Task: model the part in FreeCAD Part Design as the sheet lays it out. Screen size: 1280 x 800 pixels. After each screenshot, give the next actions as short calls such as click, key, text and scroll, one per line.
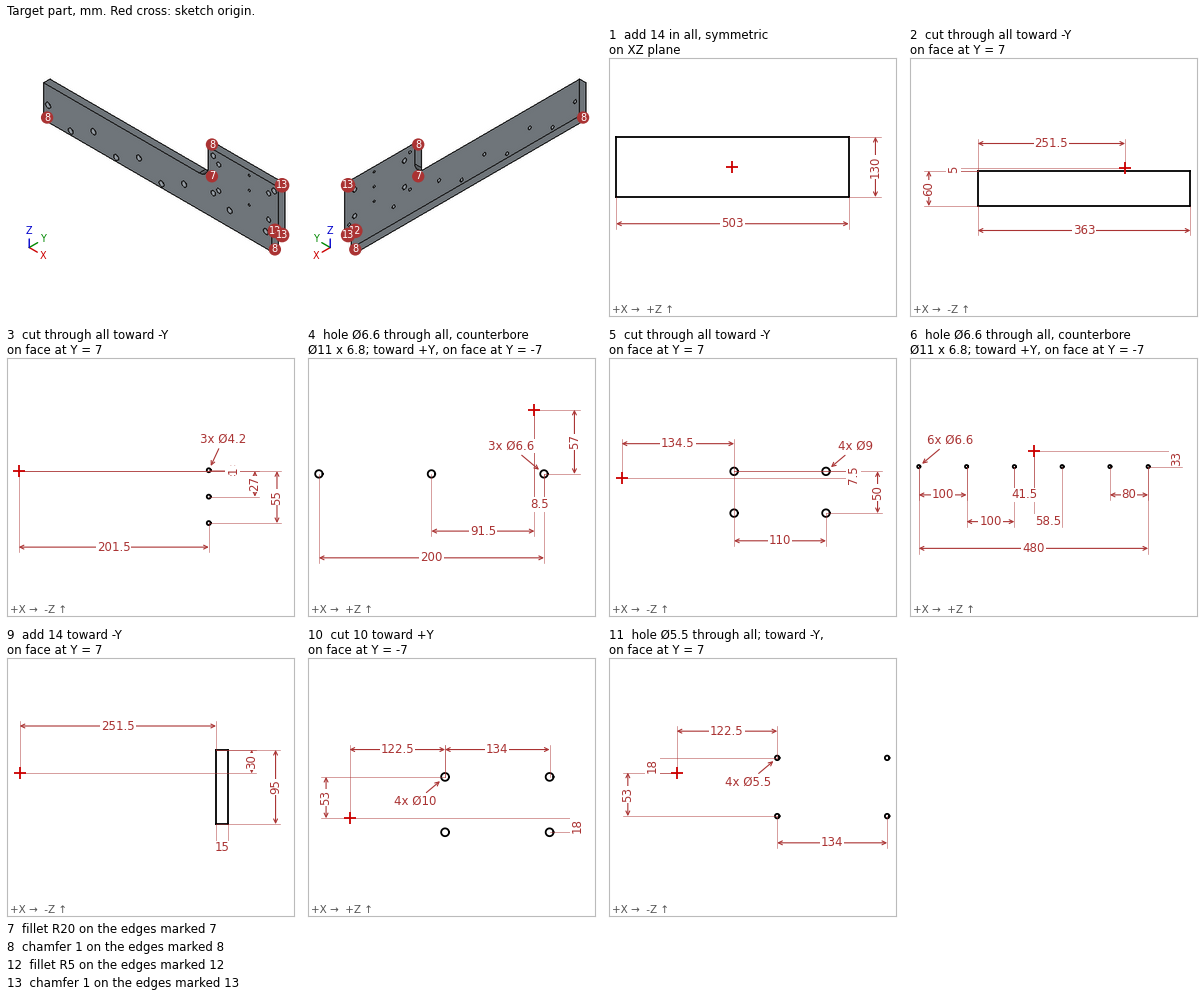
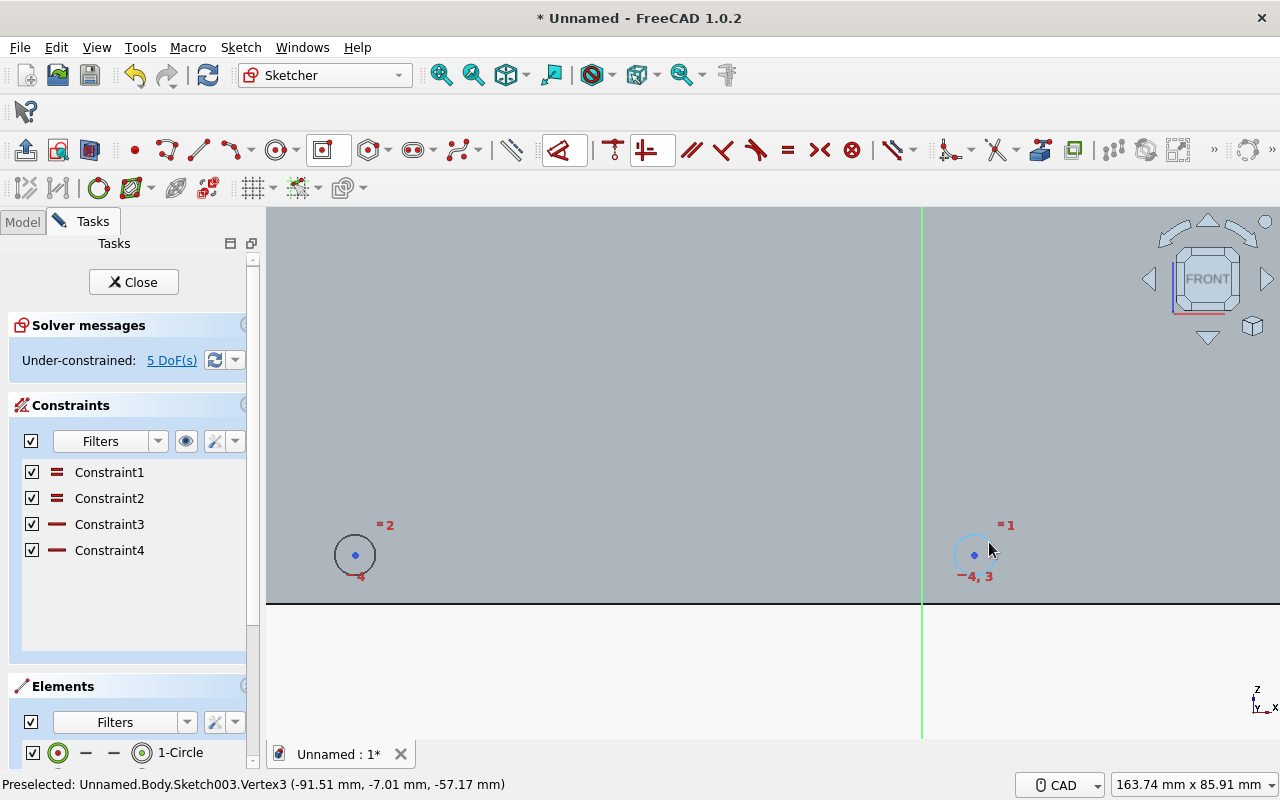
click(989, 541)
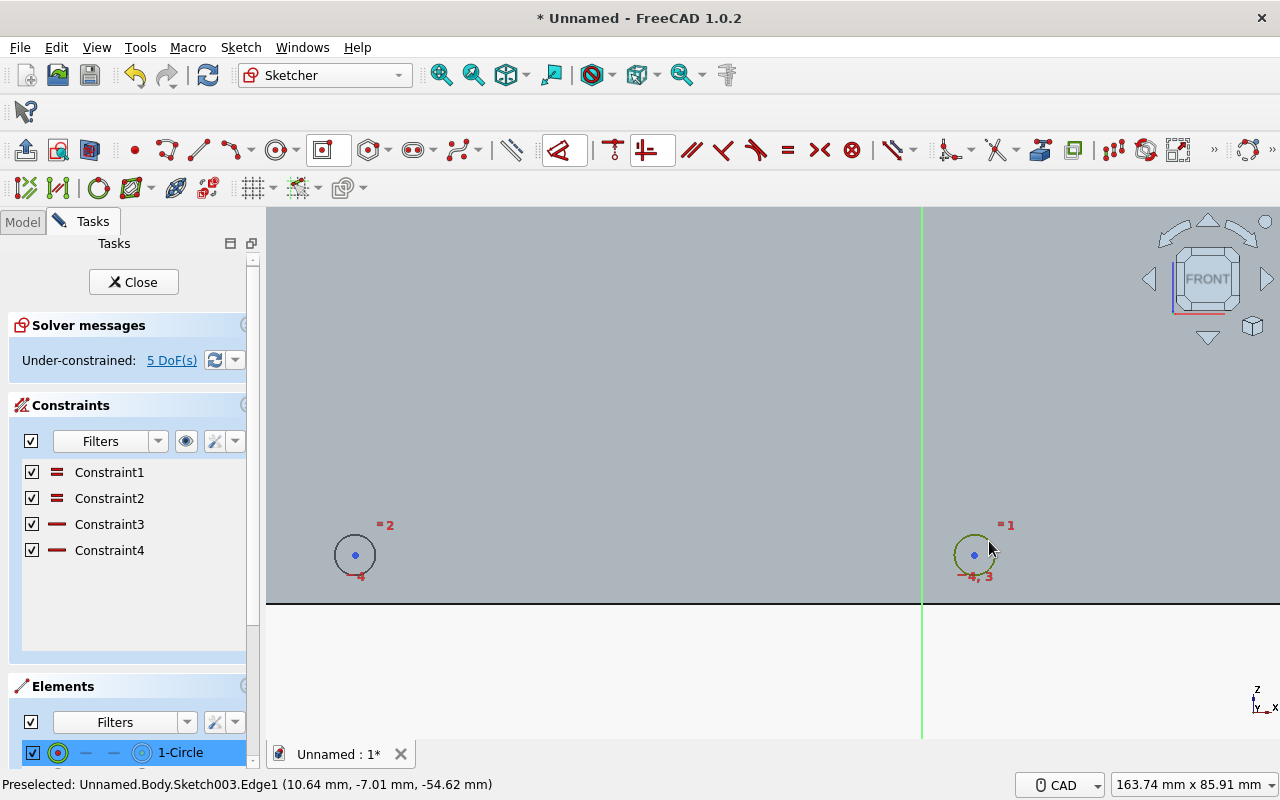
click(582, 150)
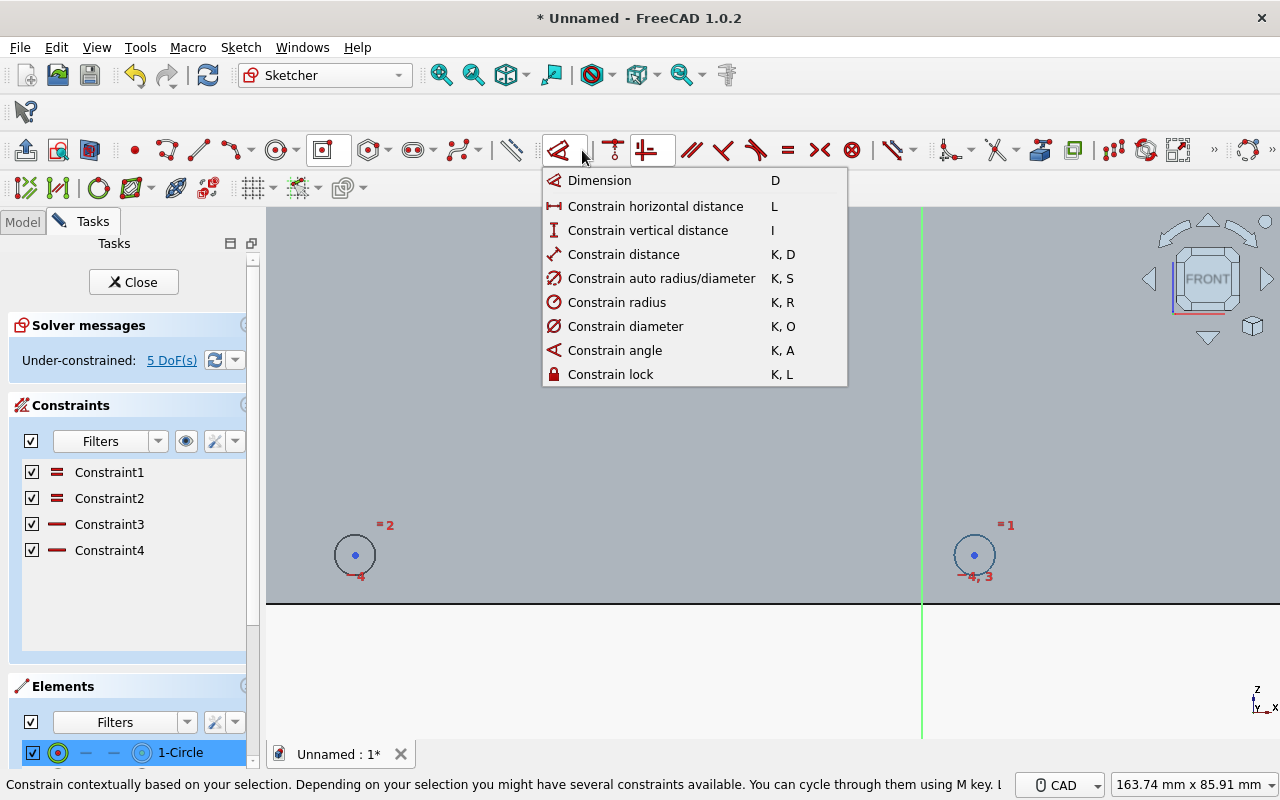
click(695, 326)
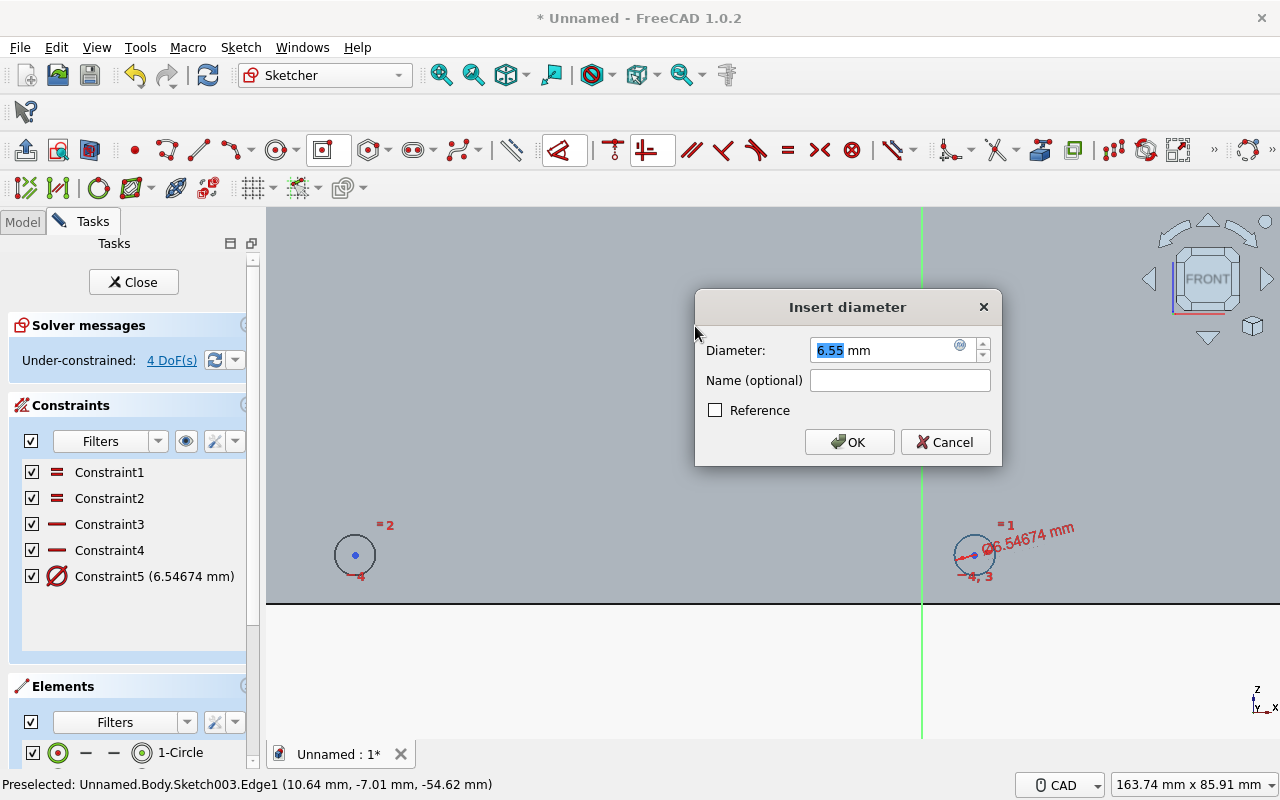
text(6.6)
key(Return)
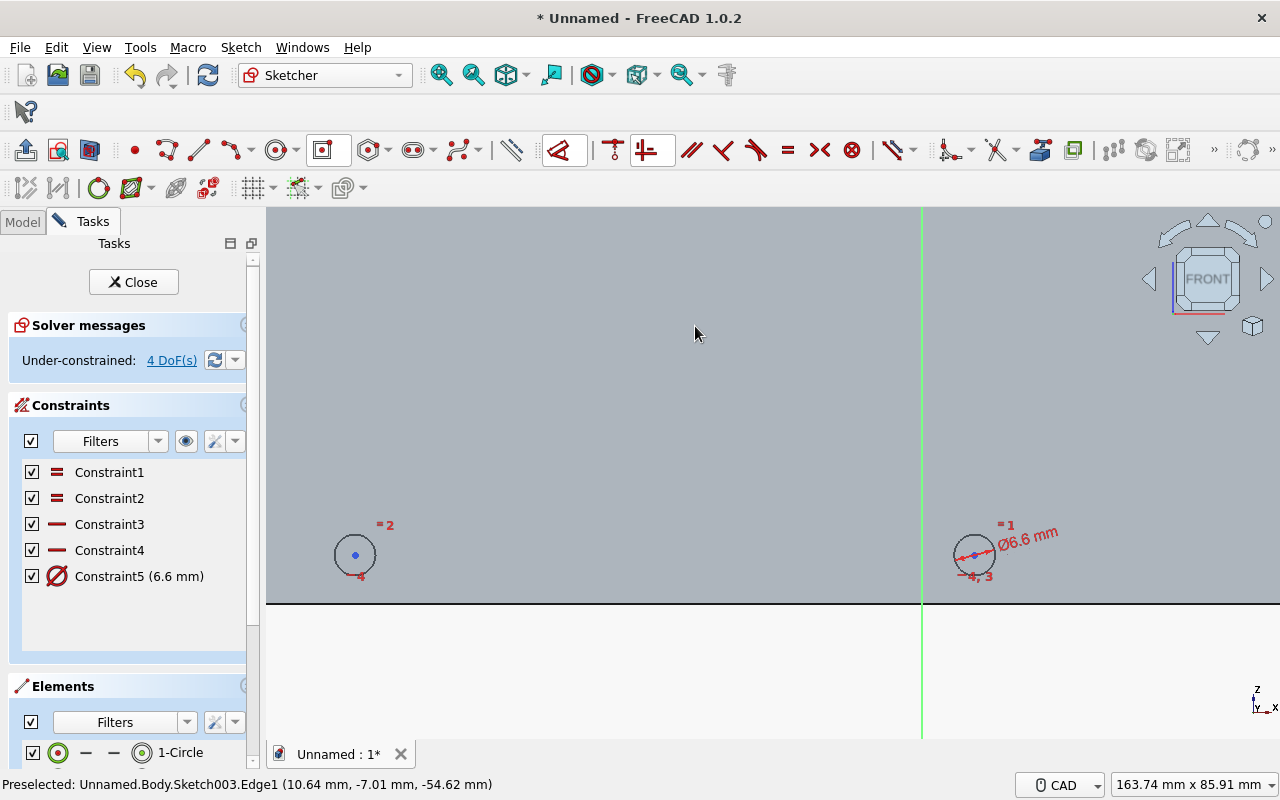
click(975, 555)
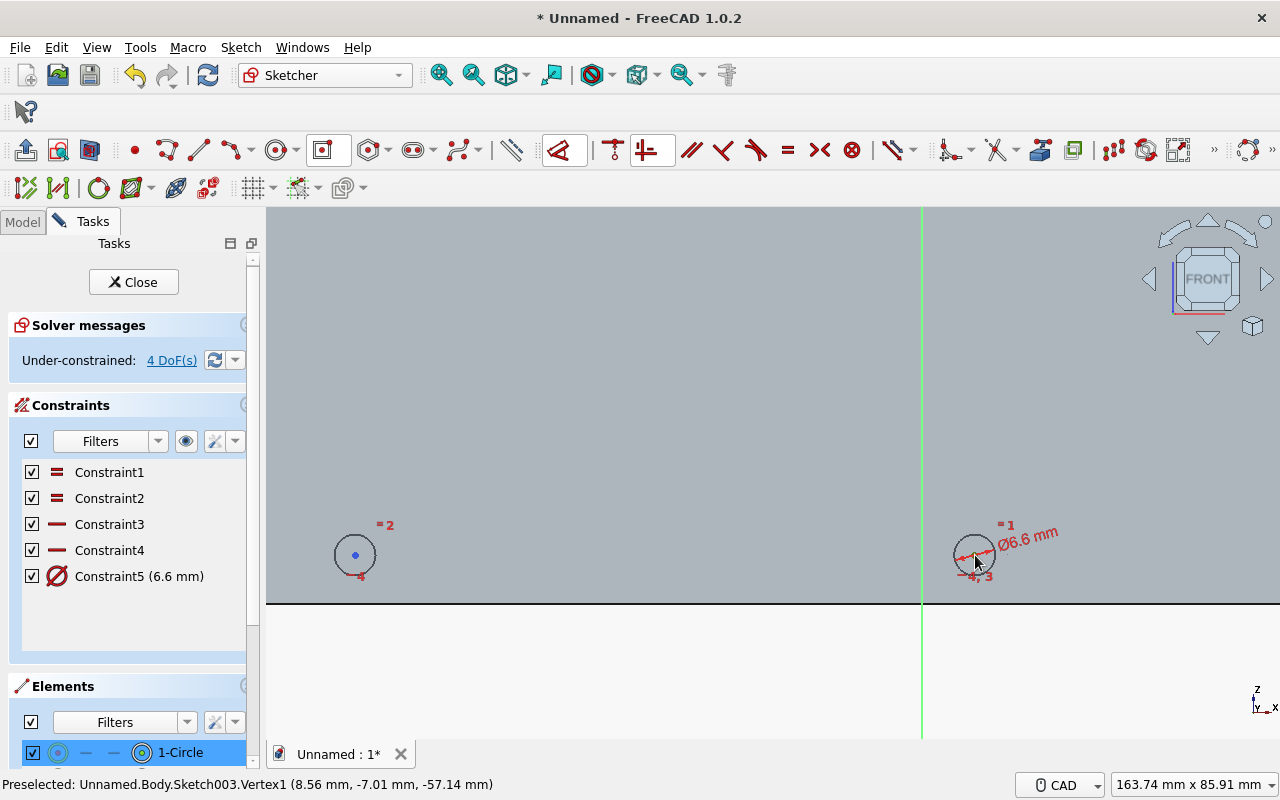
key(i)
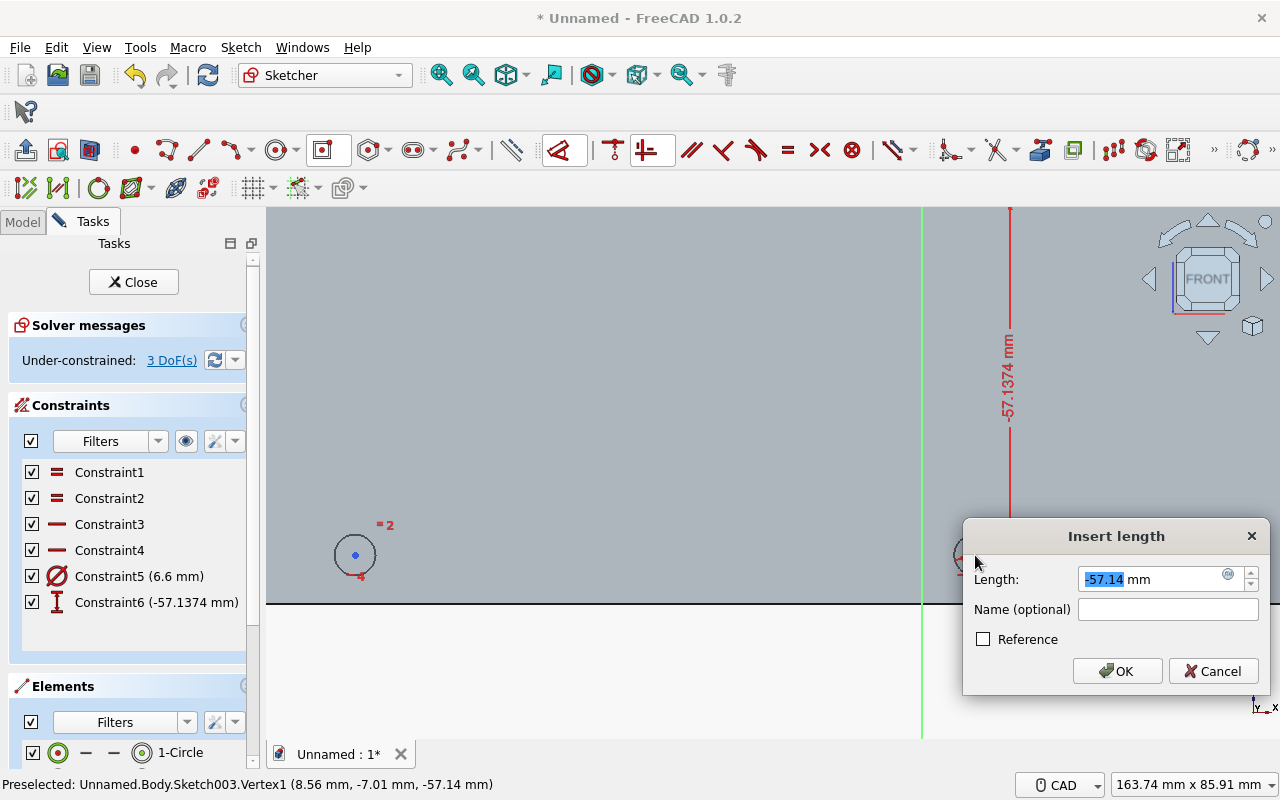
text(-57)
key(Return)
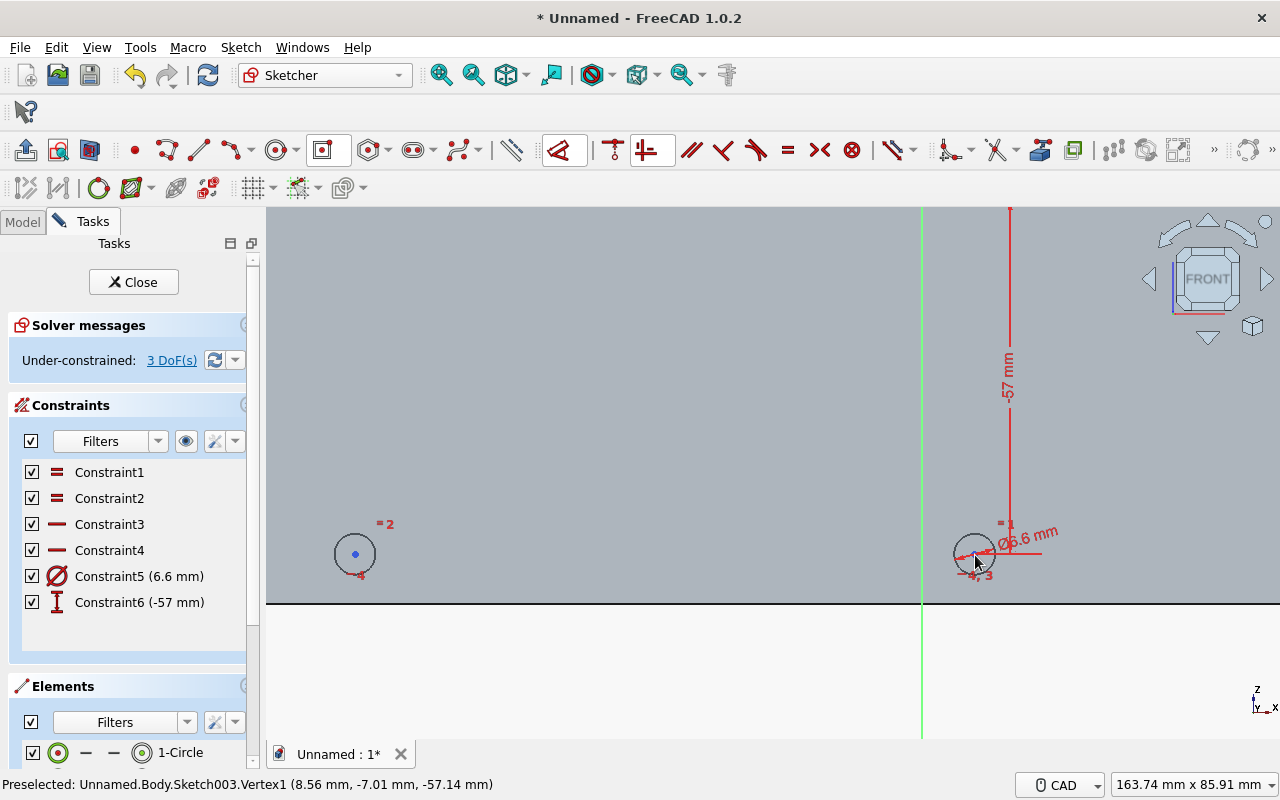
click(975, 554)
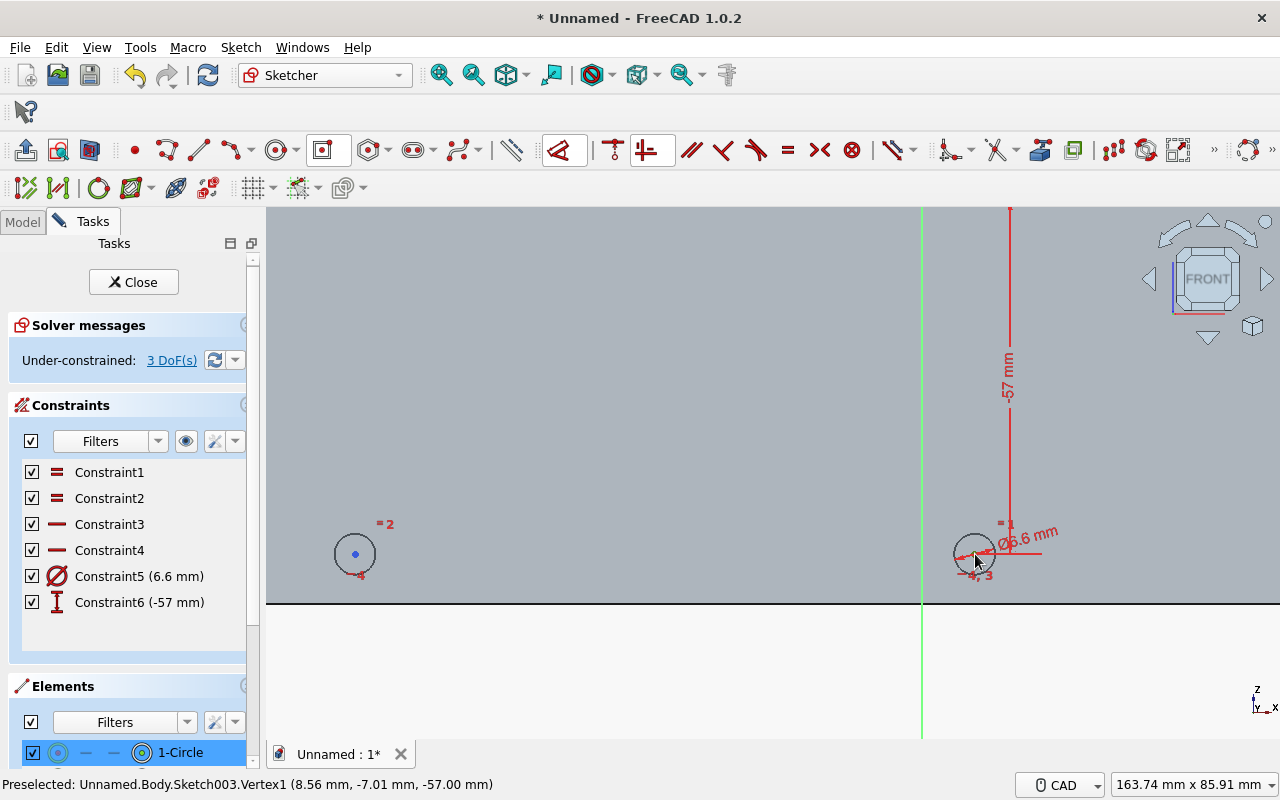
key(l)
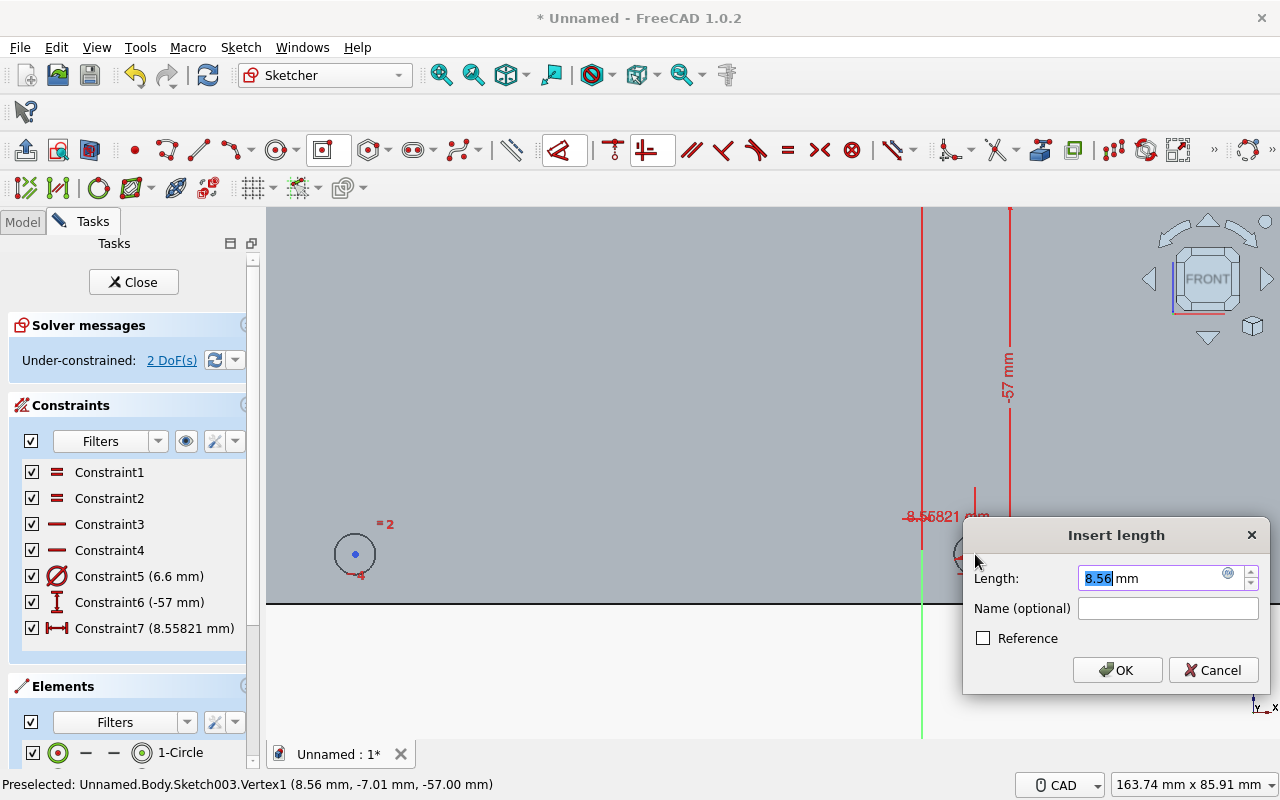
text(8.5)
key(Return)